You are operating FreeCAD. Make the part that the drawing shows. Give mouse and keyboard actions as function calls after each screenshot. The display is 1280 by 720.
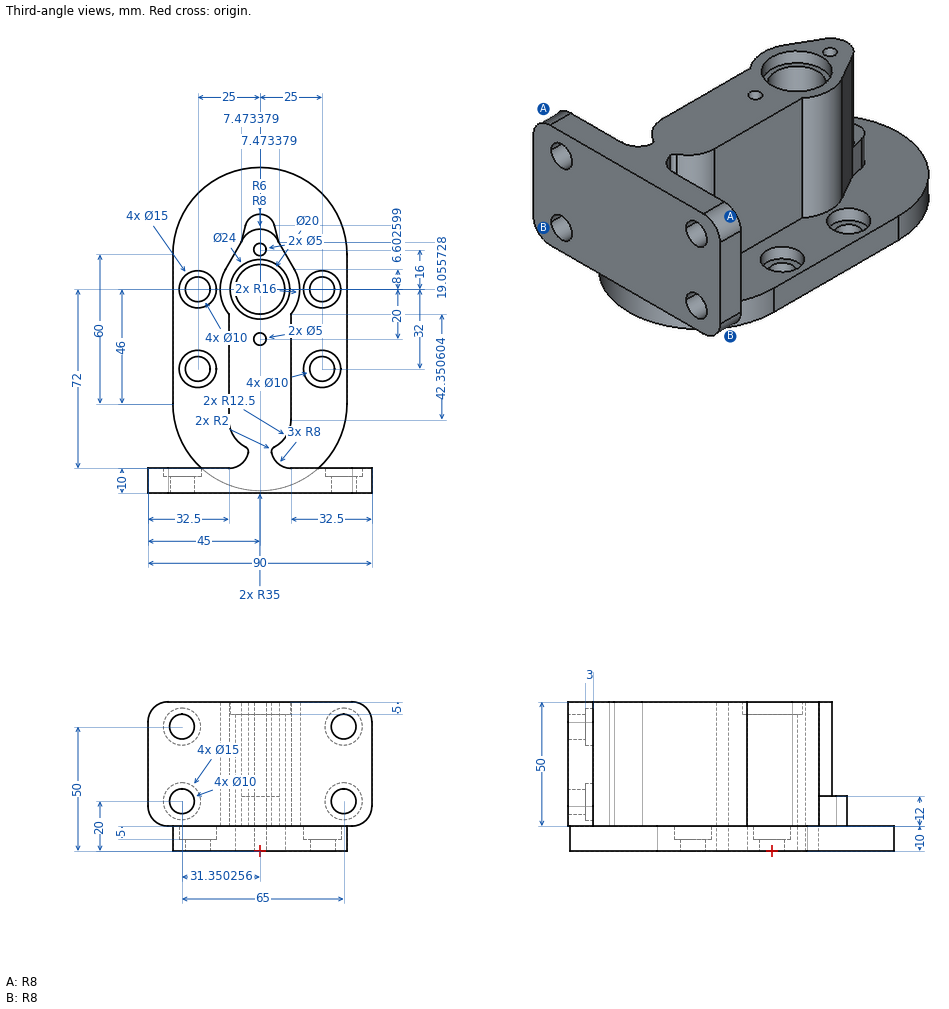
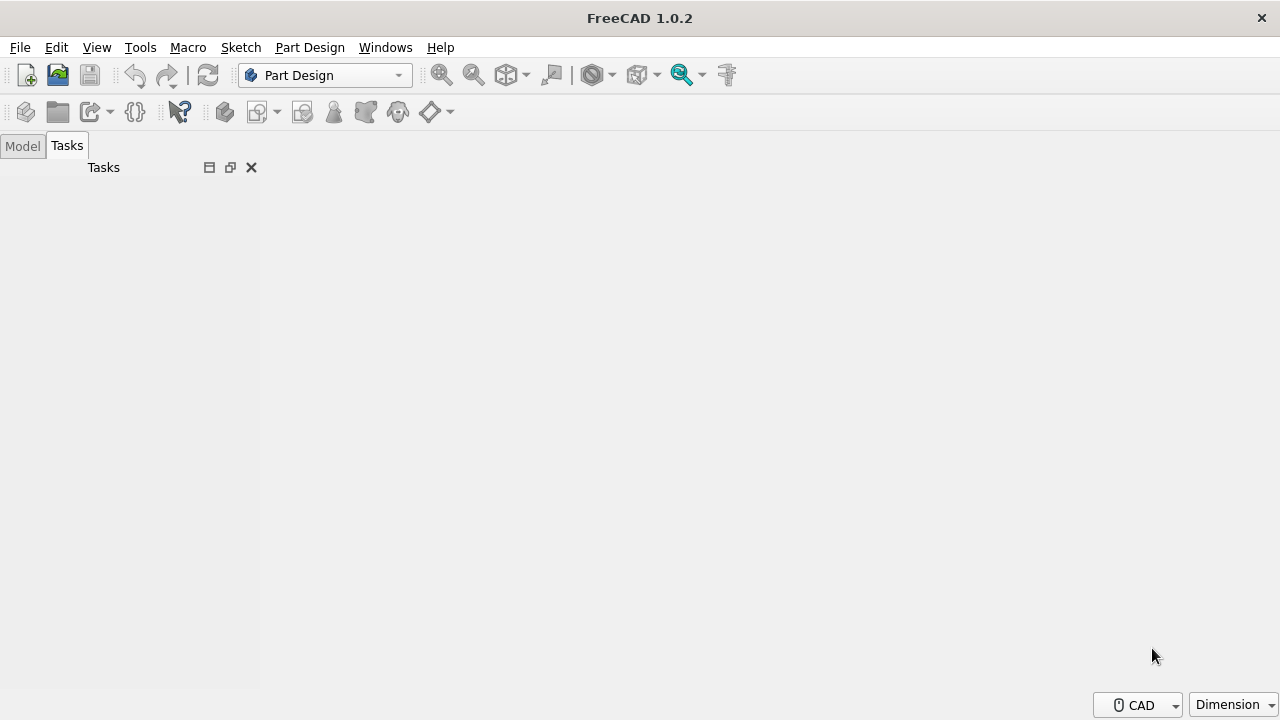
click(818, 112)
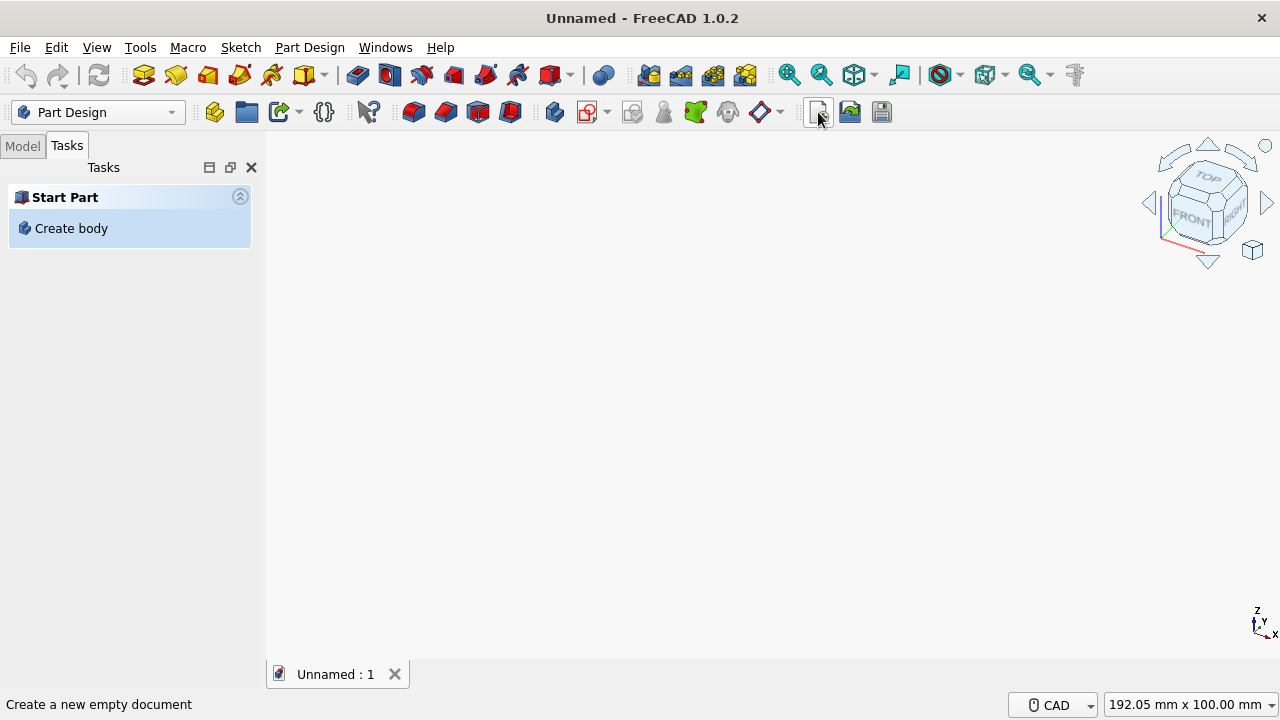
click(588, 112)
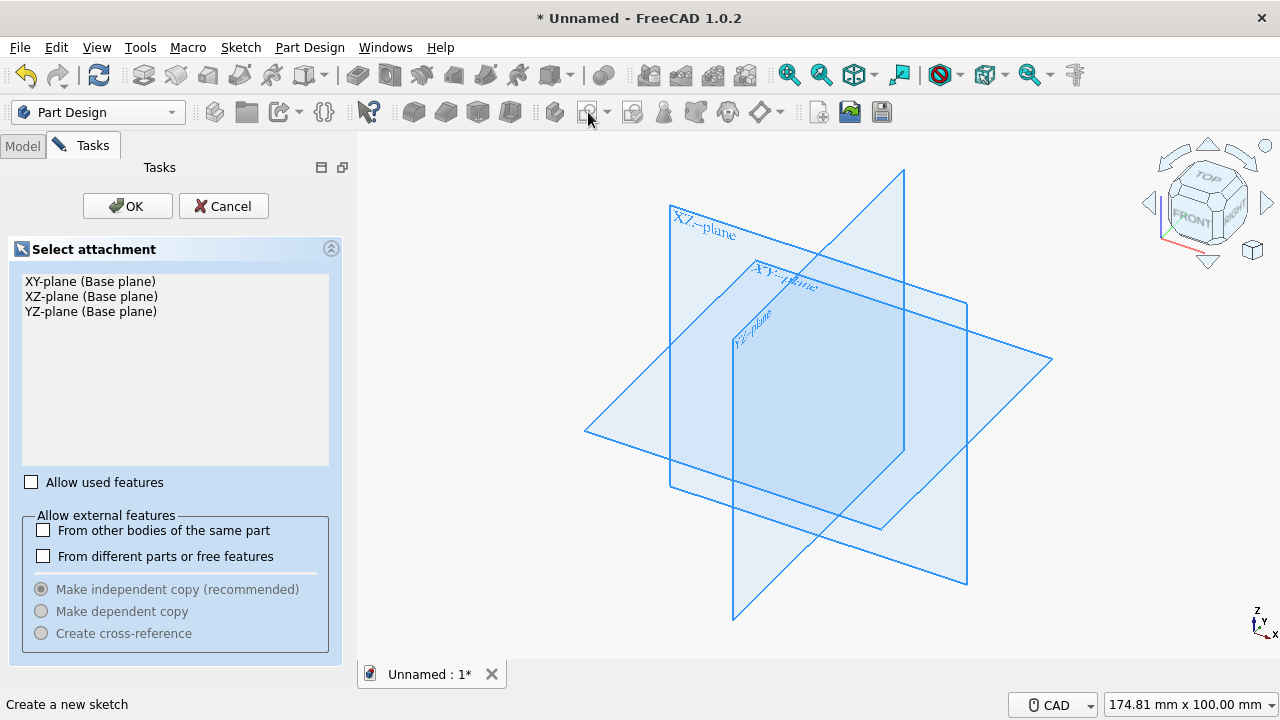
click(82, 282)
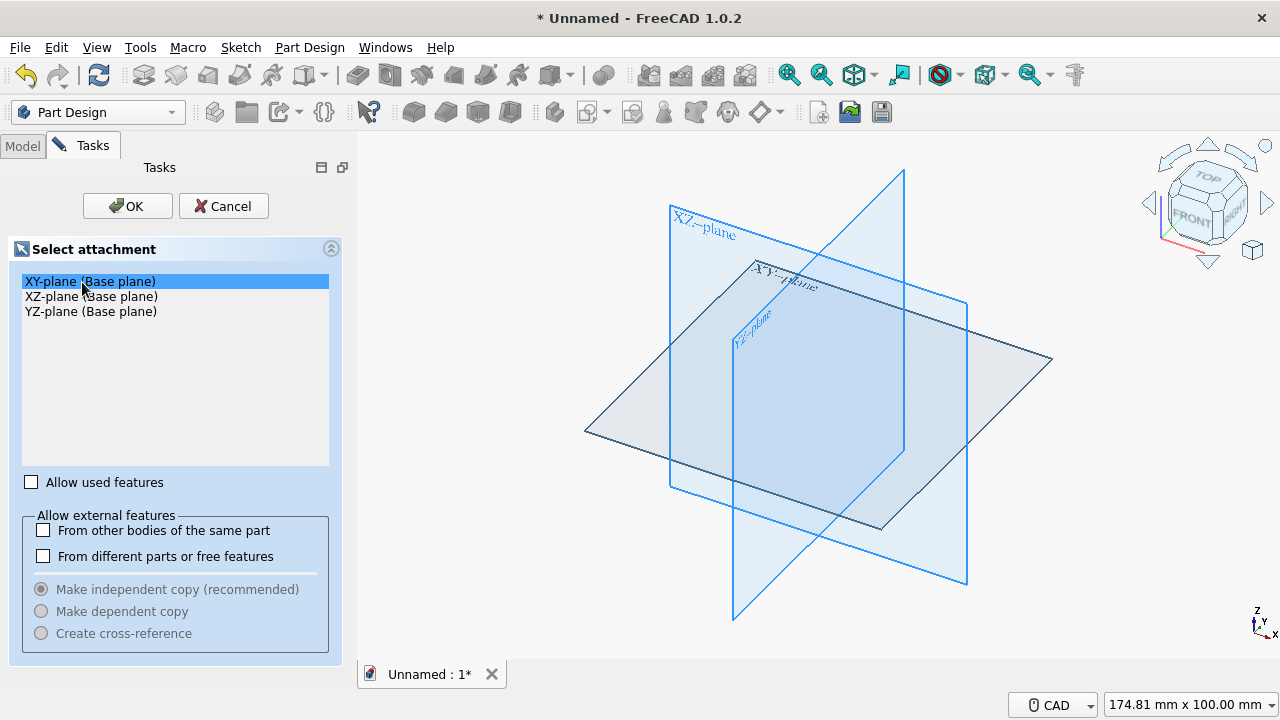
click(128, 206)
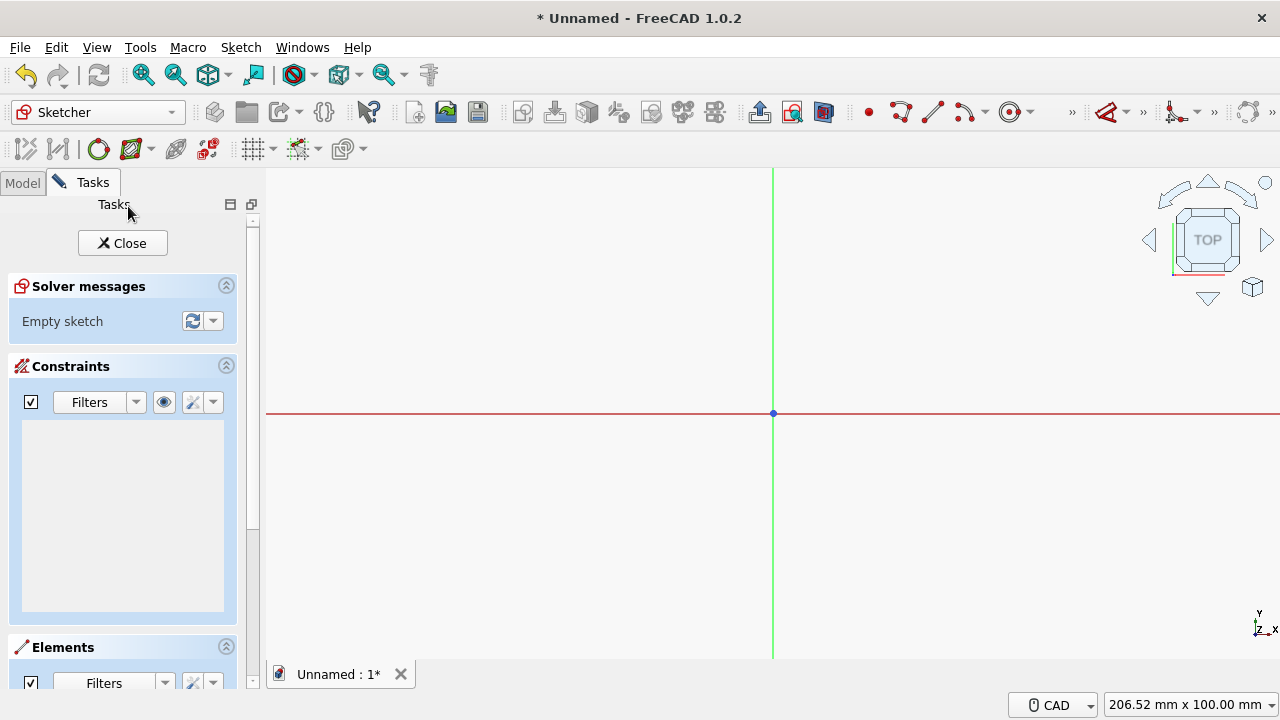
scroll(649, 349, down, 4)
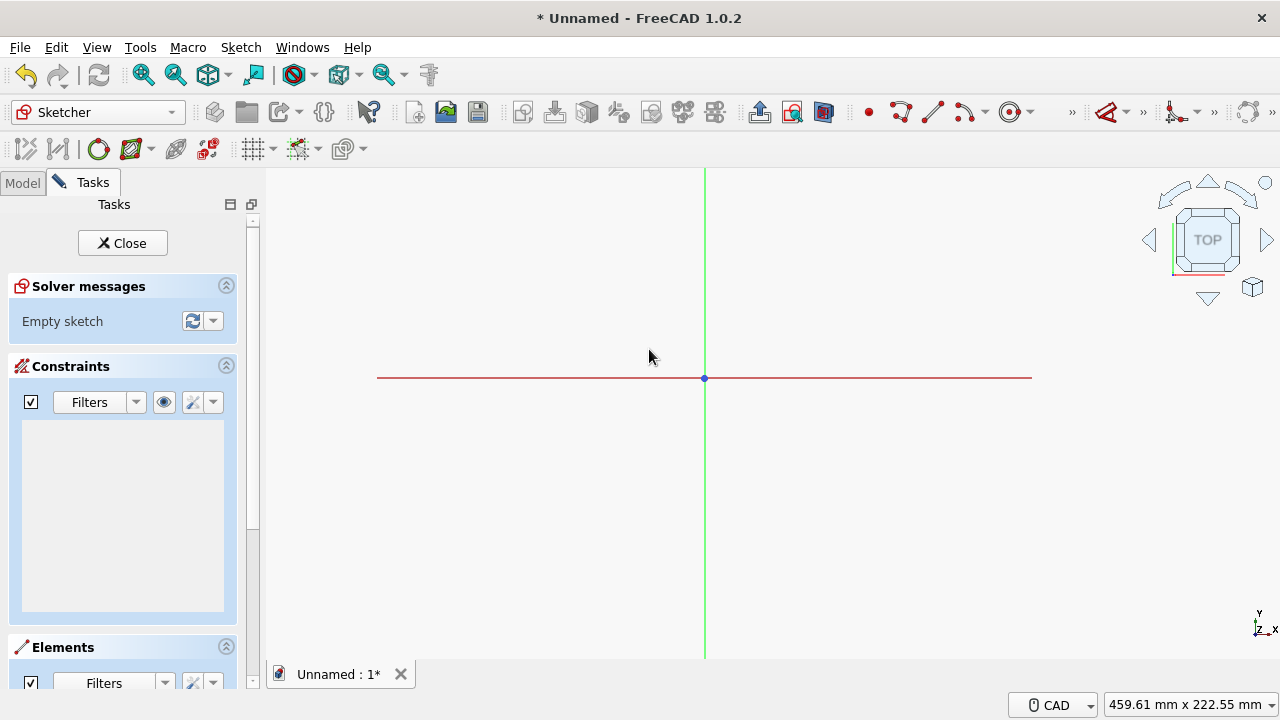
key(g)
key(s)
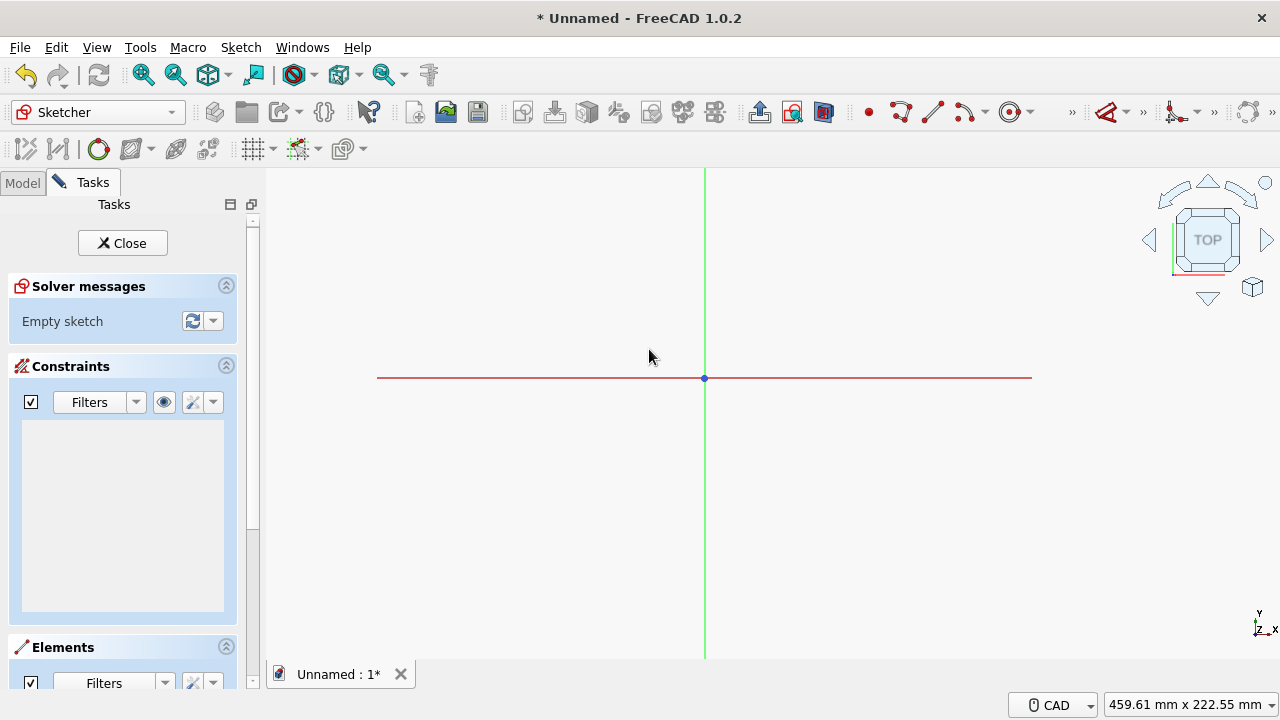
click(705, 480)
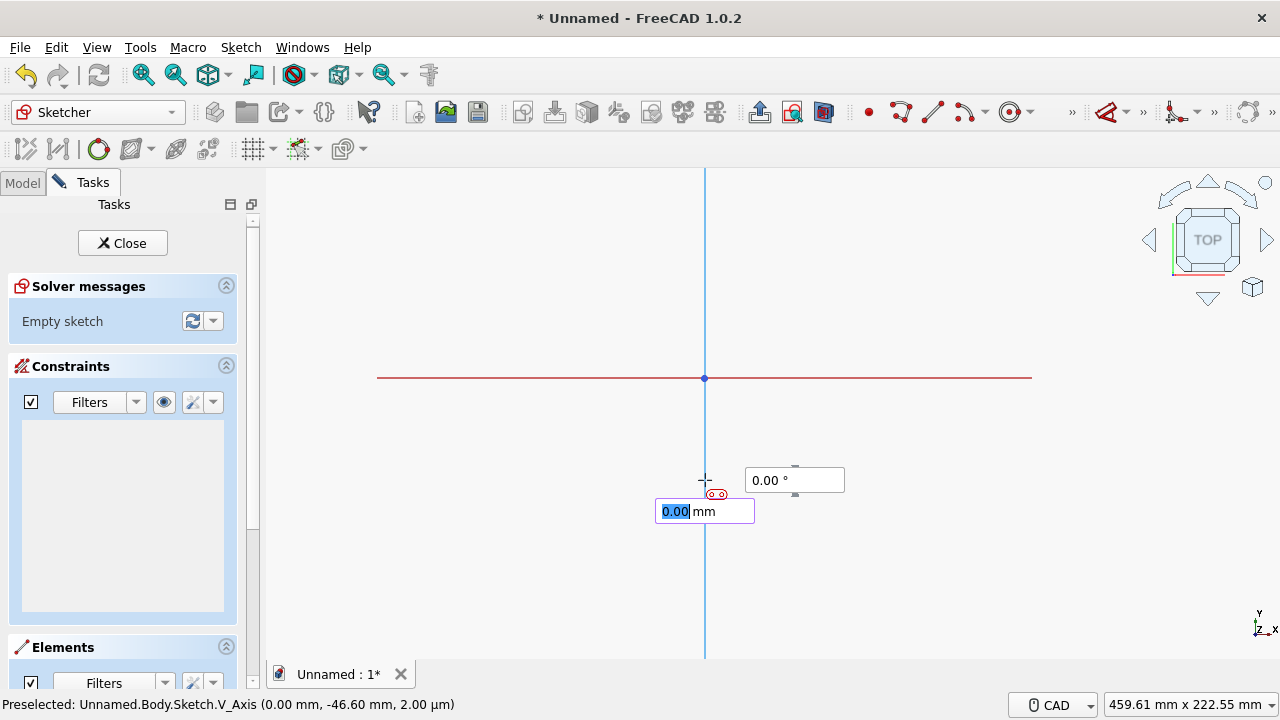
click(714, 347)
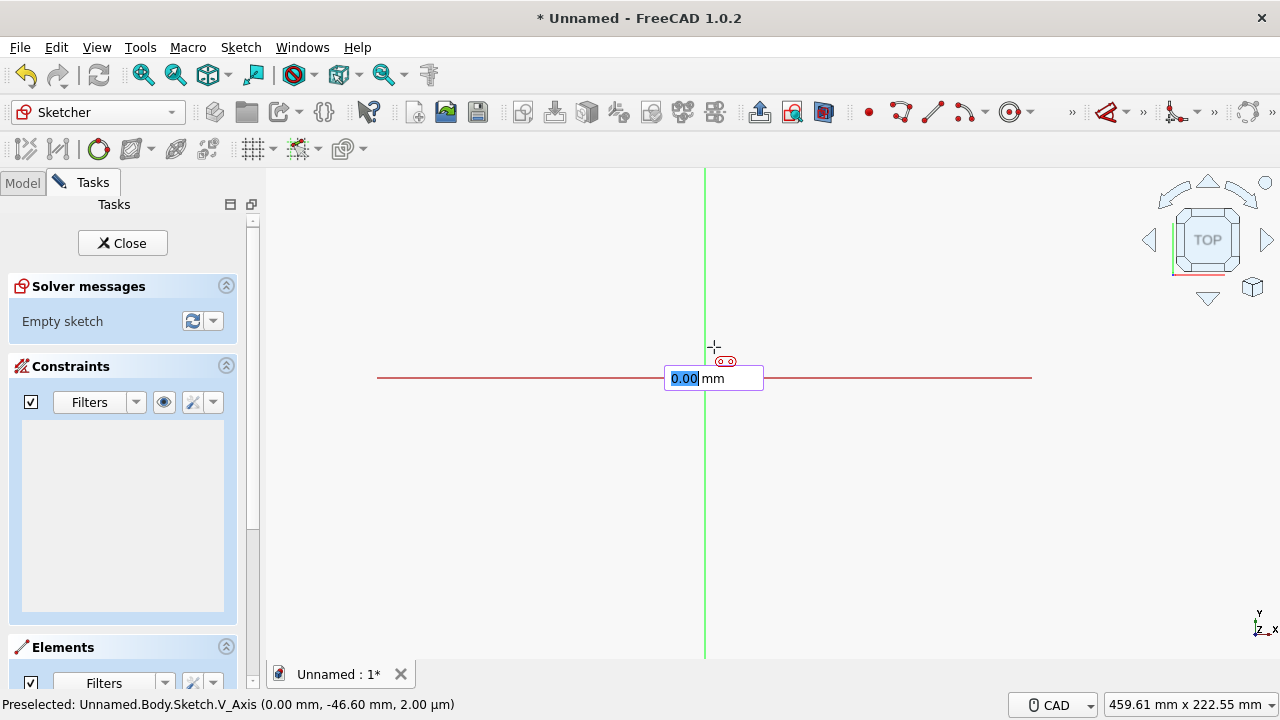
click(628, 413)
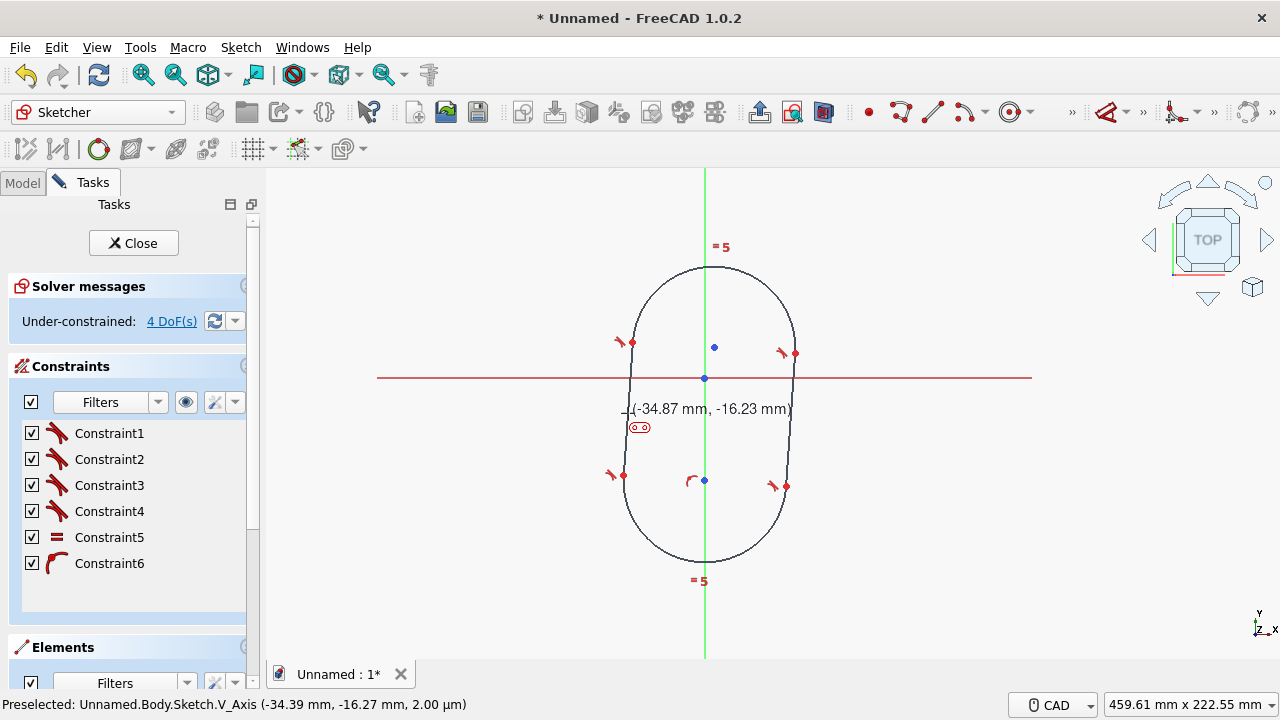
click(1010, 112)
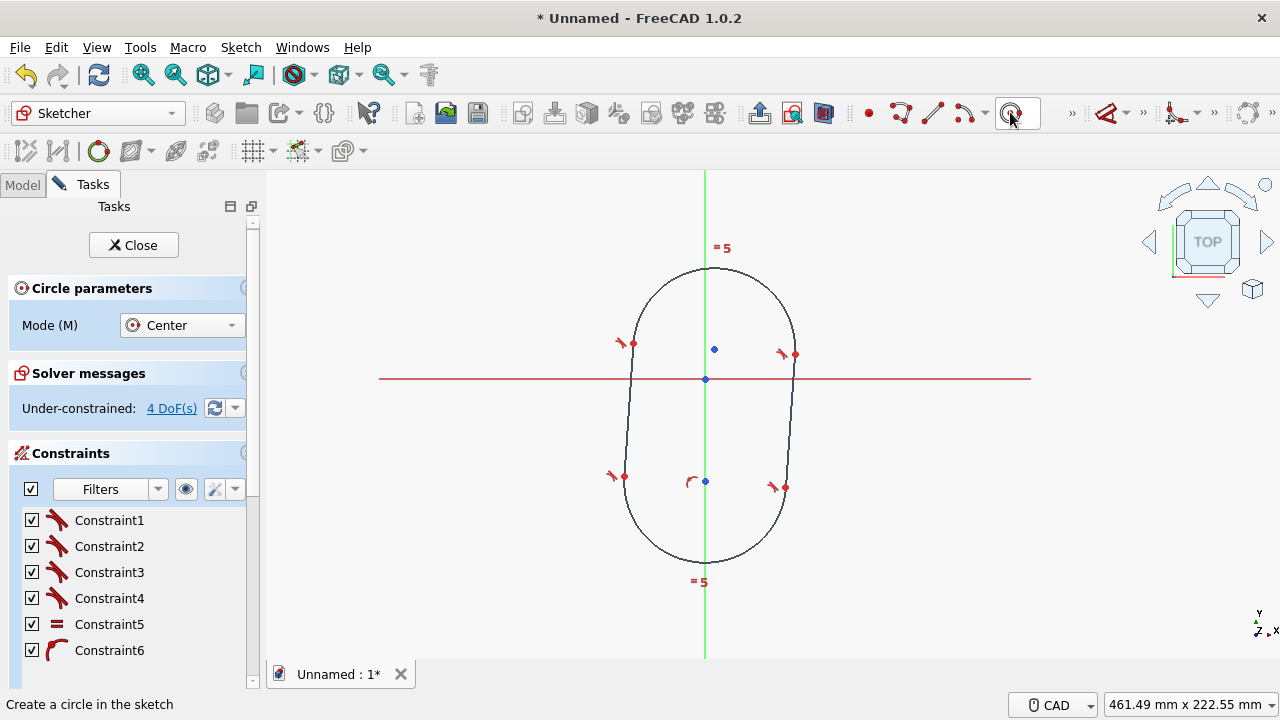
scroll(760, 450, up, 4)